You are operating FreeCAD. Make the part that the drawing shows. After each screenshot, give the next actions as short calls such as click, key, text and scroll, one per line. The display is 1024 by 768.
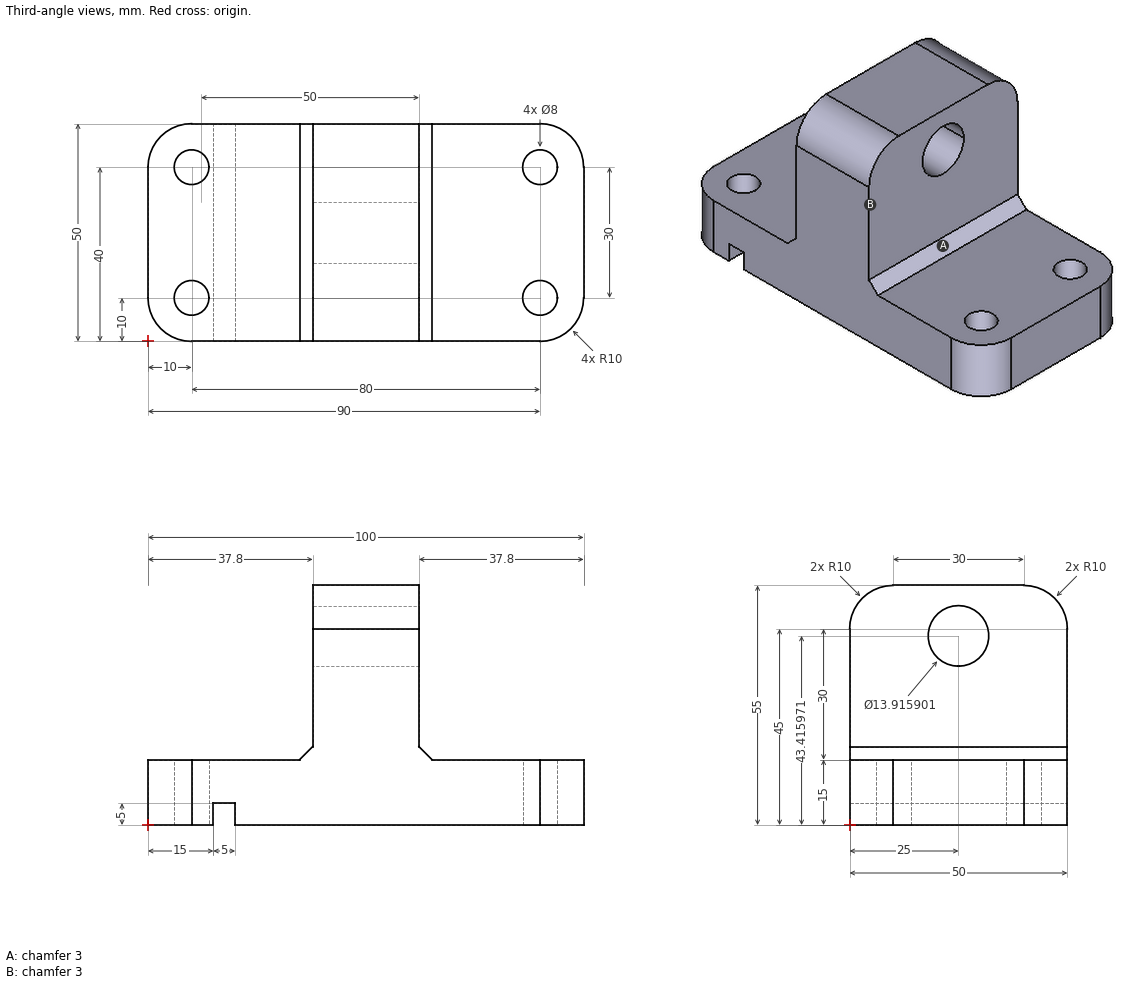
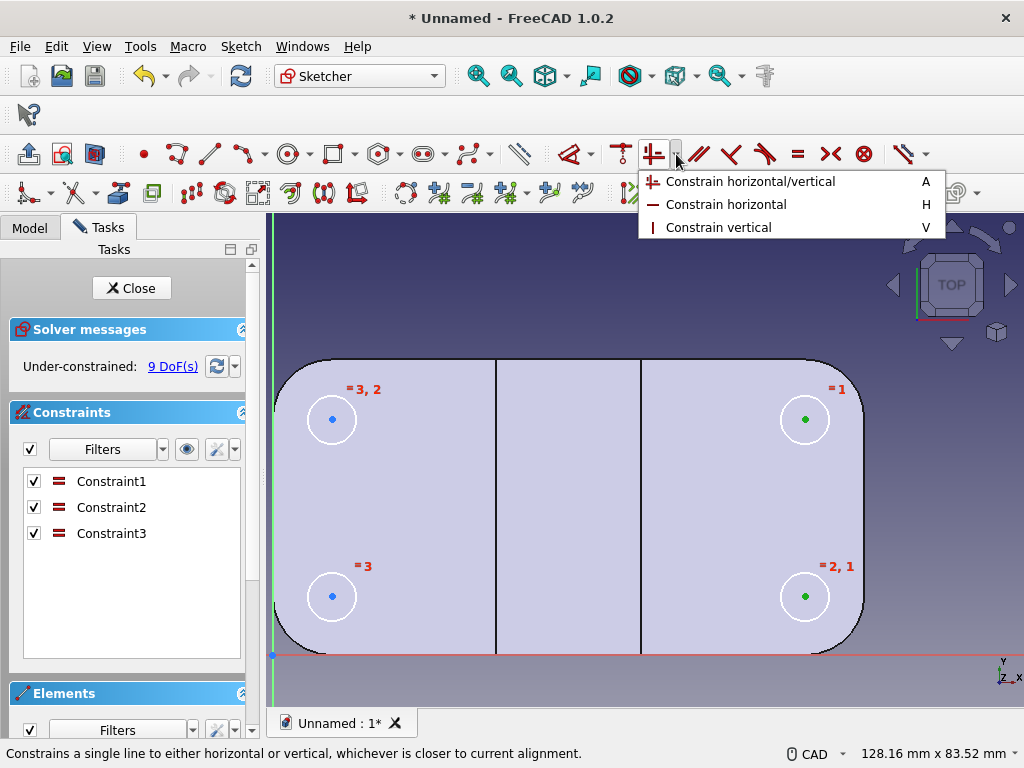
click(792, 228)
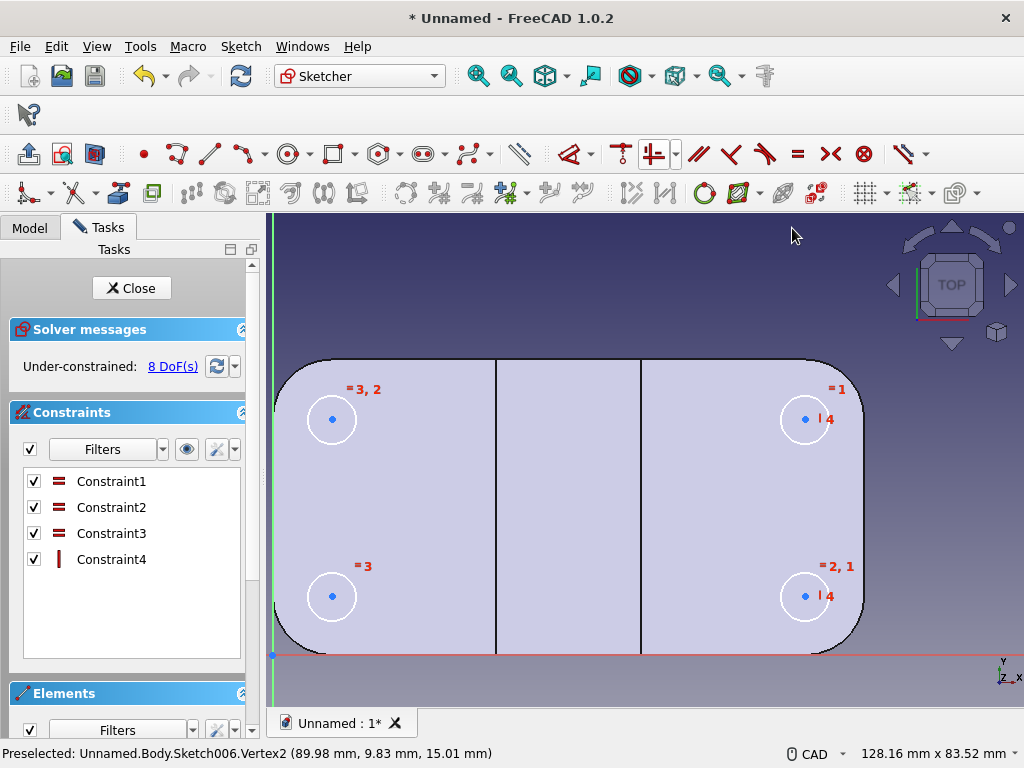
click(805, 420)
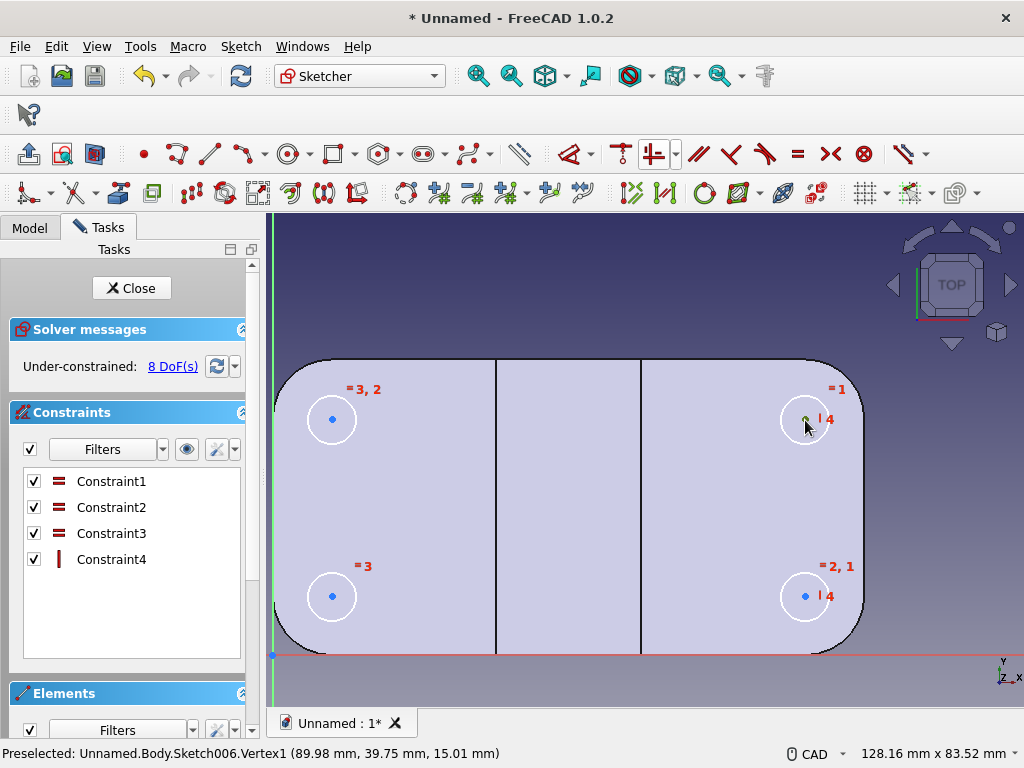
click(332, 420)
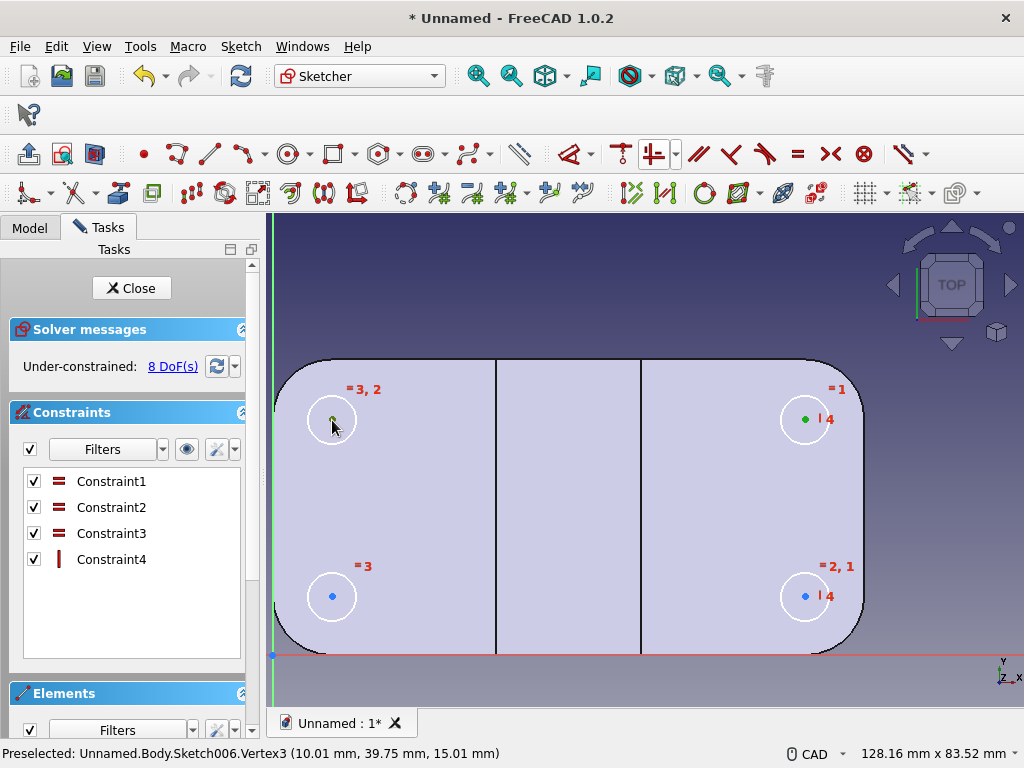
click(676, 154)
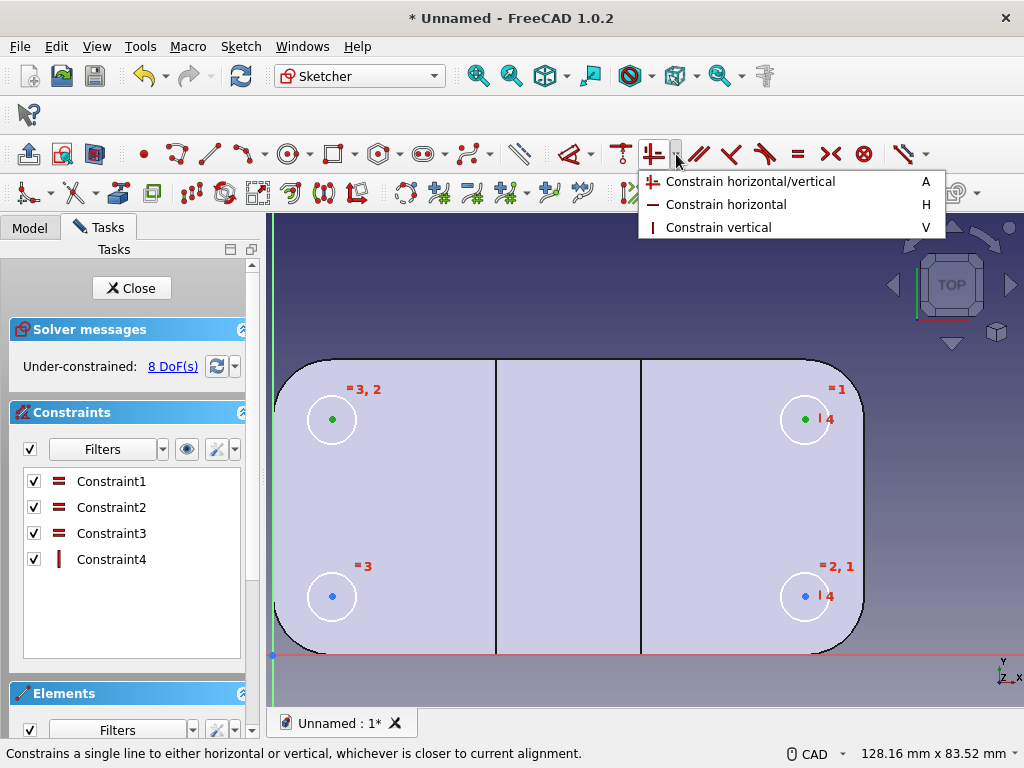
click(792, 204)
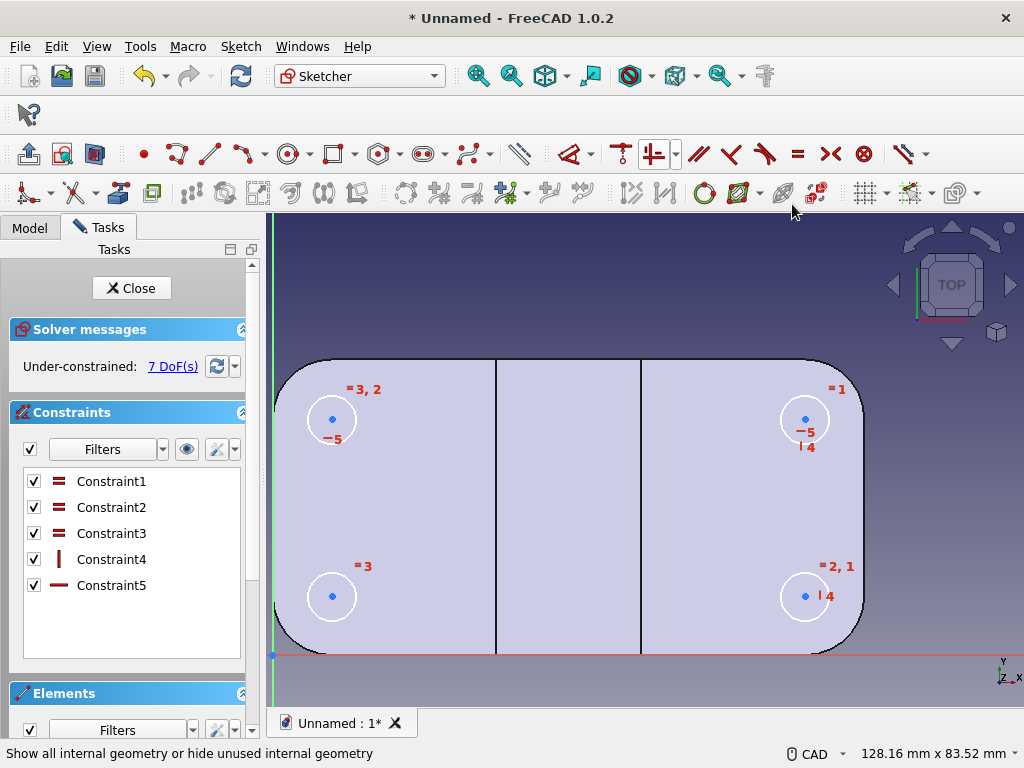
click(332, 420)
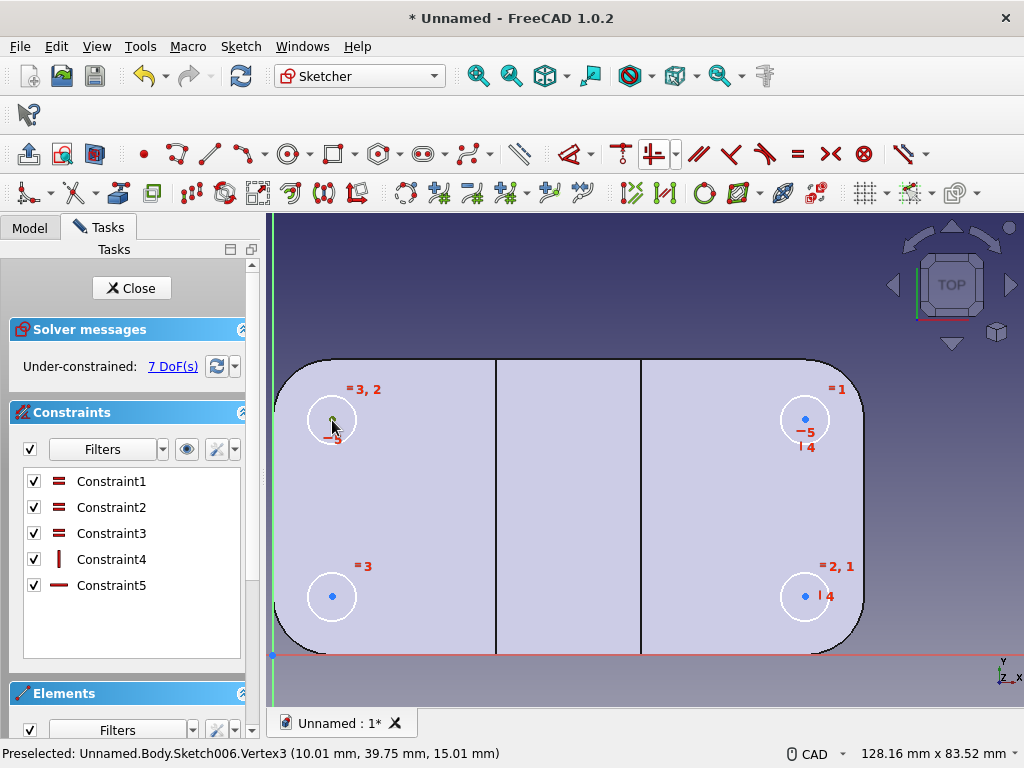
click(332, 597)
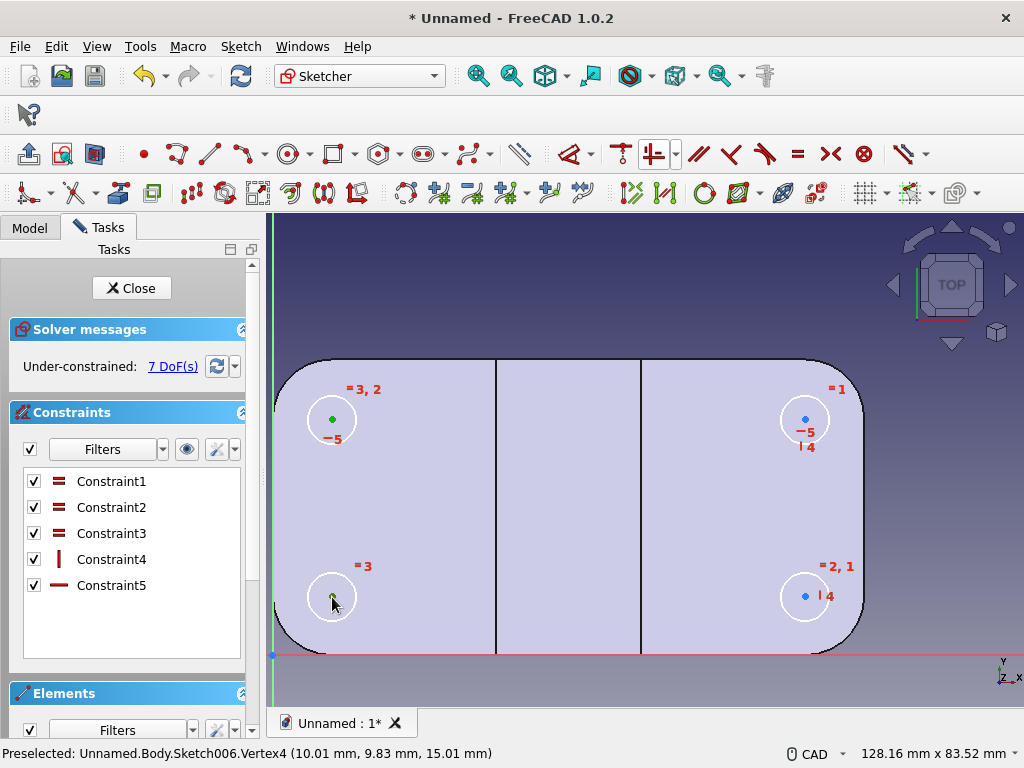
key(v)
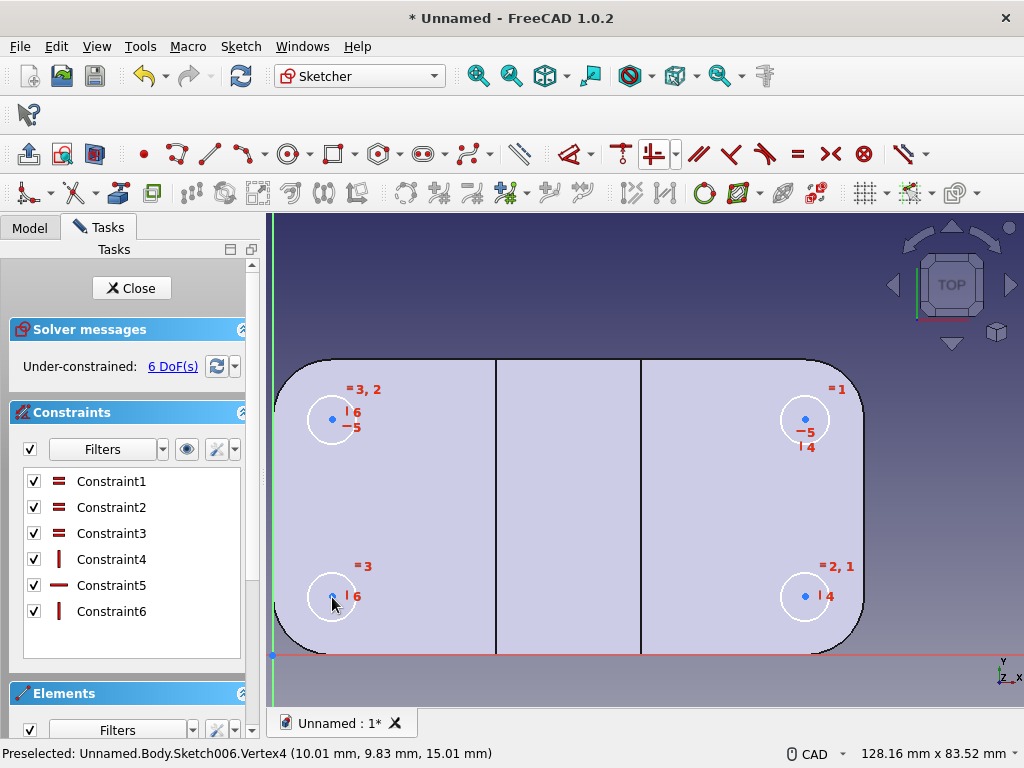
click(805, 597)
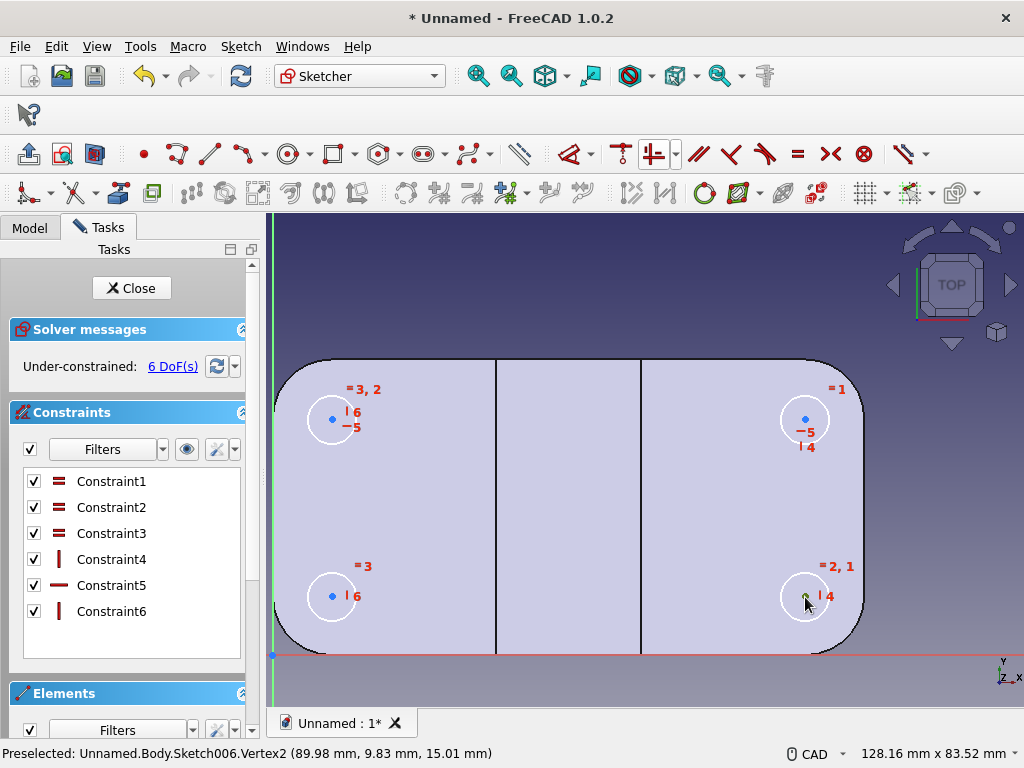
click(332, 597)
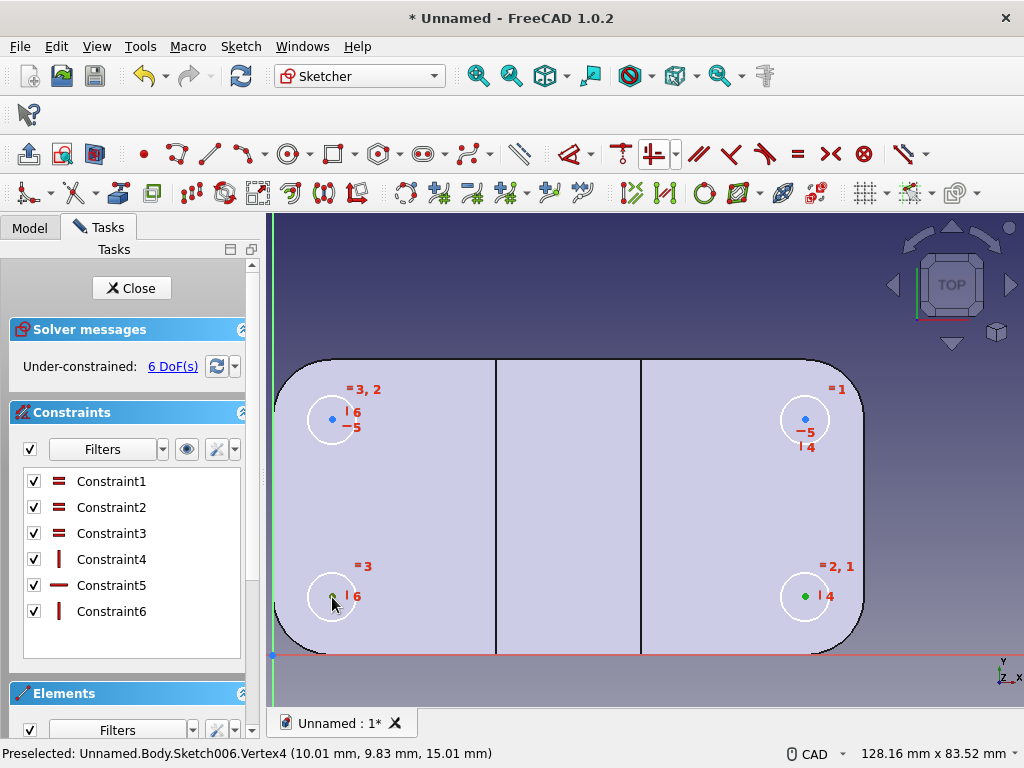
key(h)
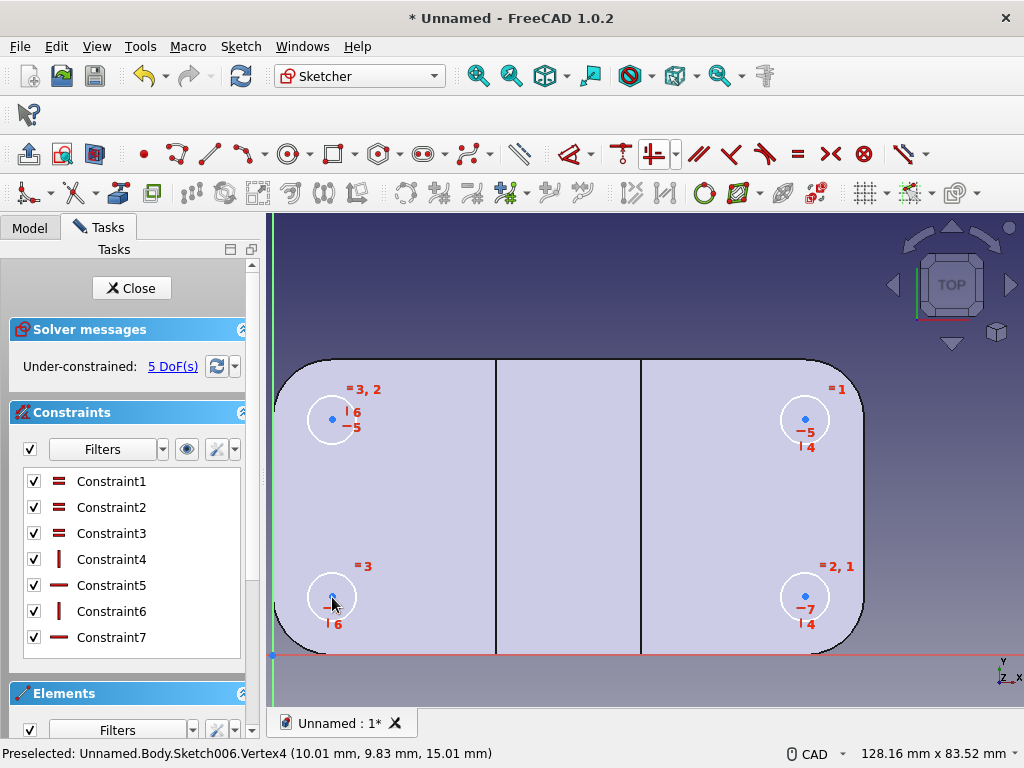
click(568, 154)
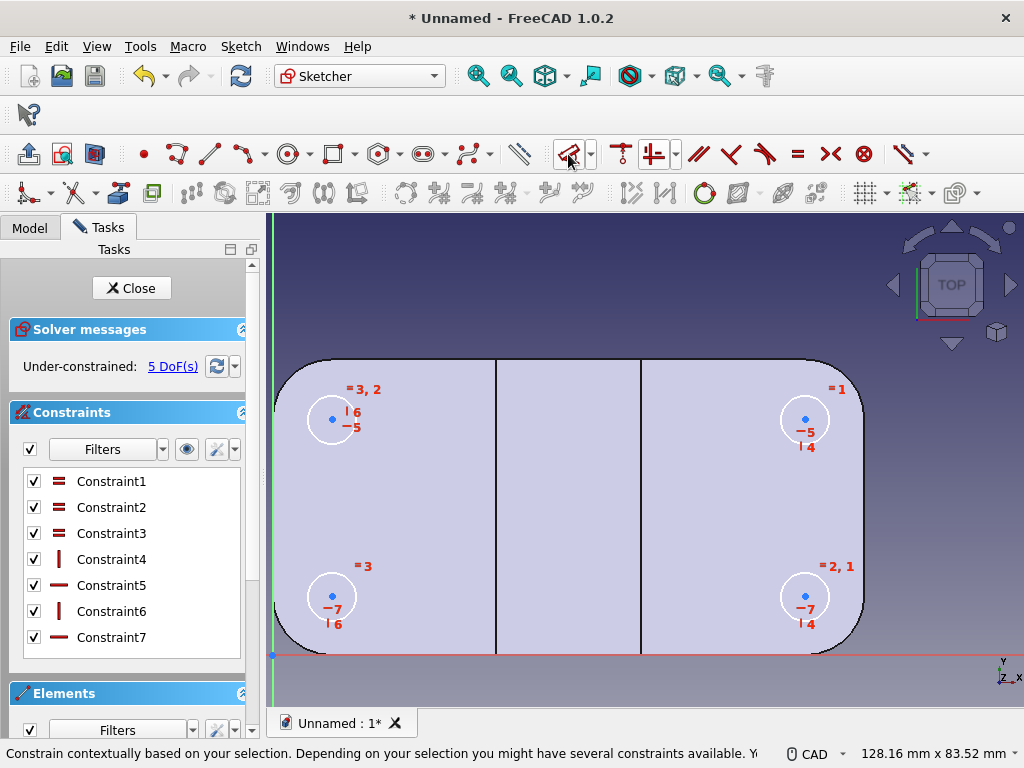
click(822, 403)
click(845, 380)